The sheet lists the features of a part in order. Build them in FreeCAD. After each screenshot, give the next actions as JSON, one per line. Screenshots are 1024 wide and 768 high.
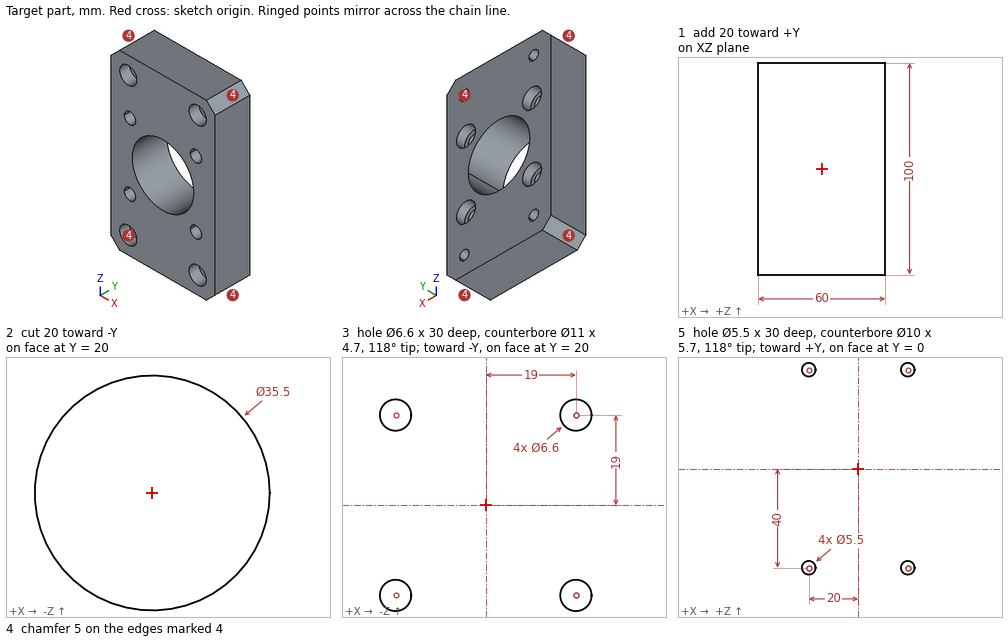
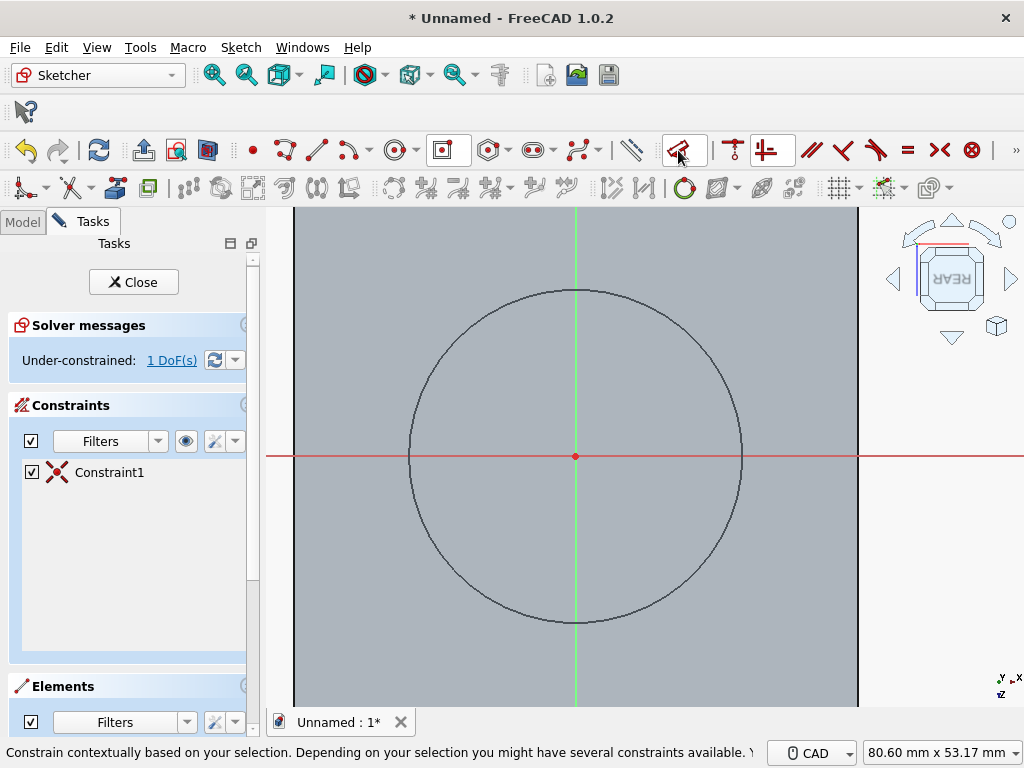
{"action": "left_click", "coordinate": [693, 338]}
{"action": "left_click", "coordinate": [716, 315]}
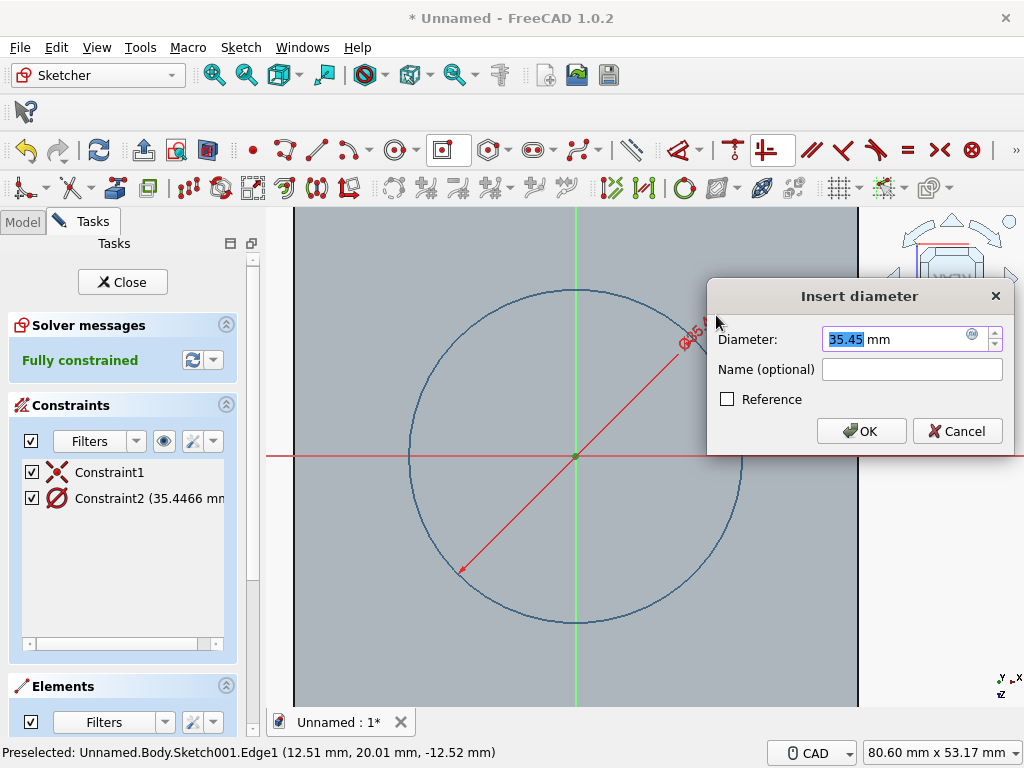
{"action": "type", "text": "35.5"}
{"action": "key", "text": "Return"}
{"action": "key", "text": "Escape"}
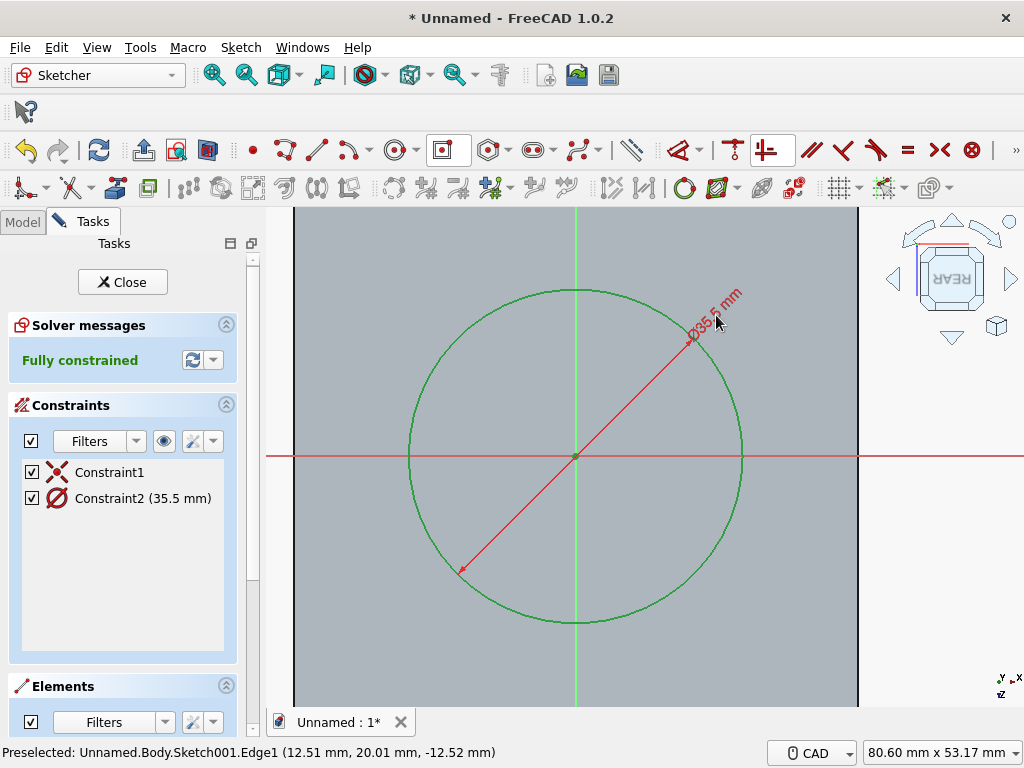
{"action": "left_click", "coordinate": [123, 282]}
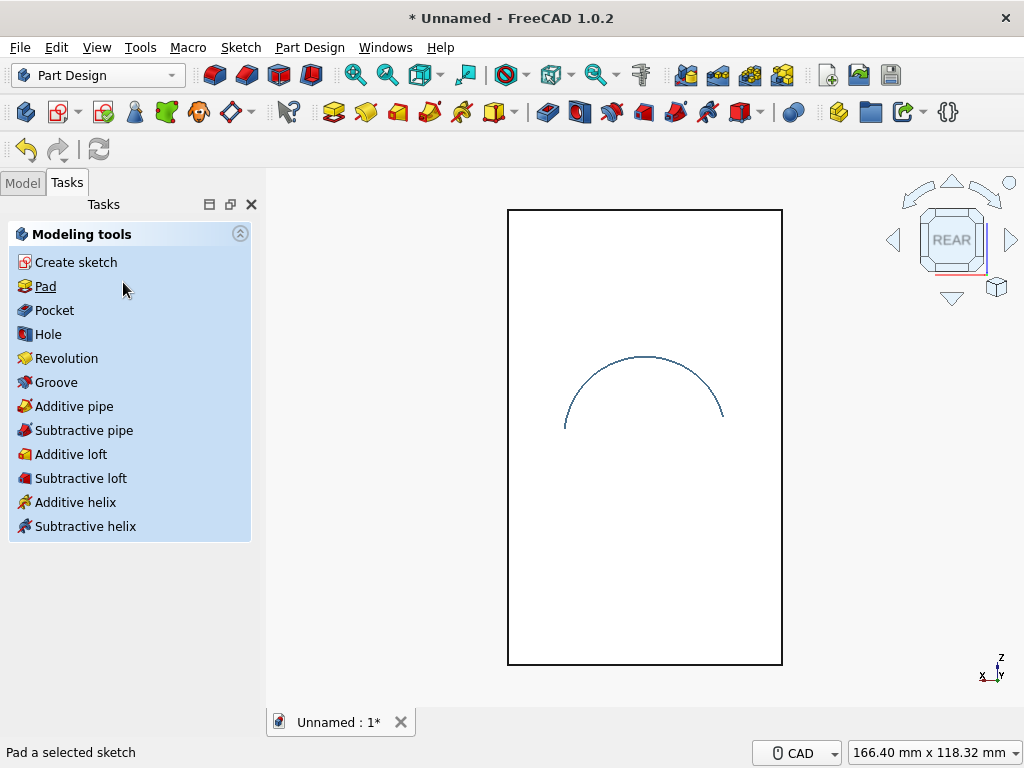
{"action": "left_click", "coordinate": [548, 112]}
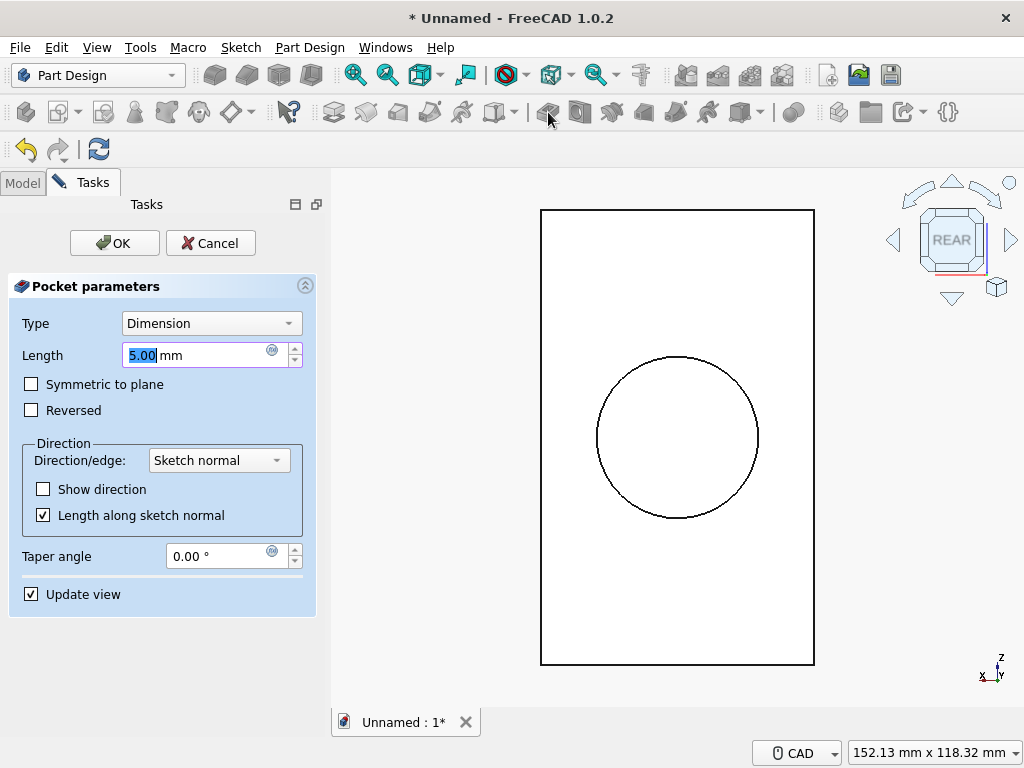
{"action": "type", "text": "20"}
{"action": "key", "text": "Tab"}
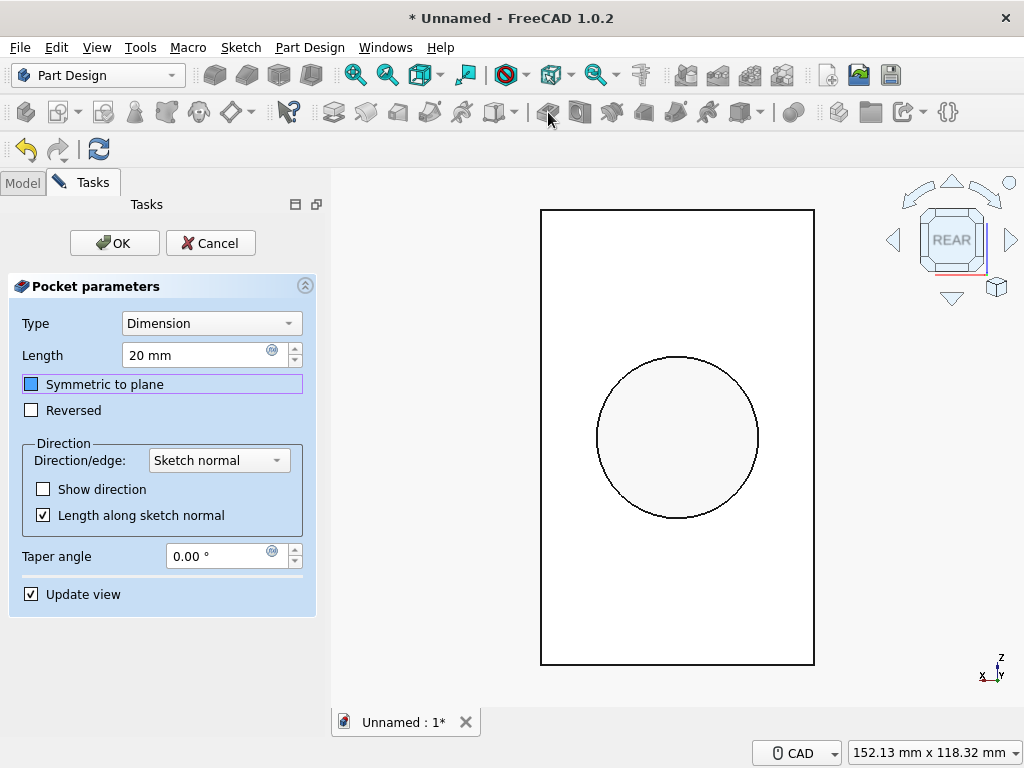
{"action": "left_click", "coordinate": [115, 243]}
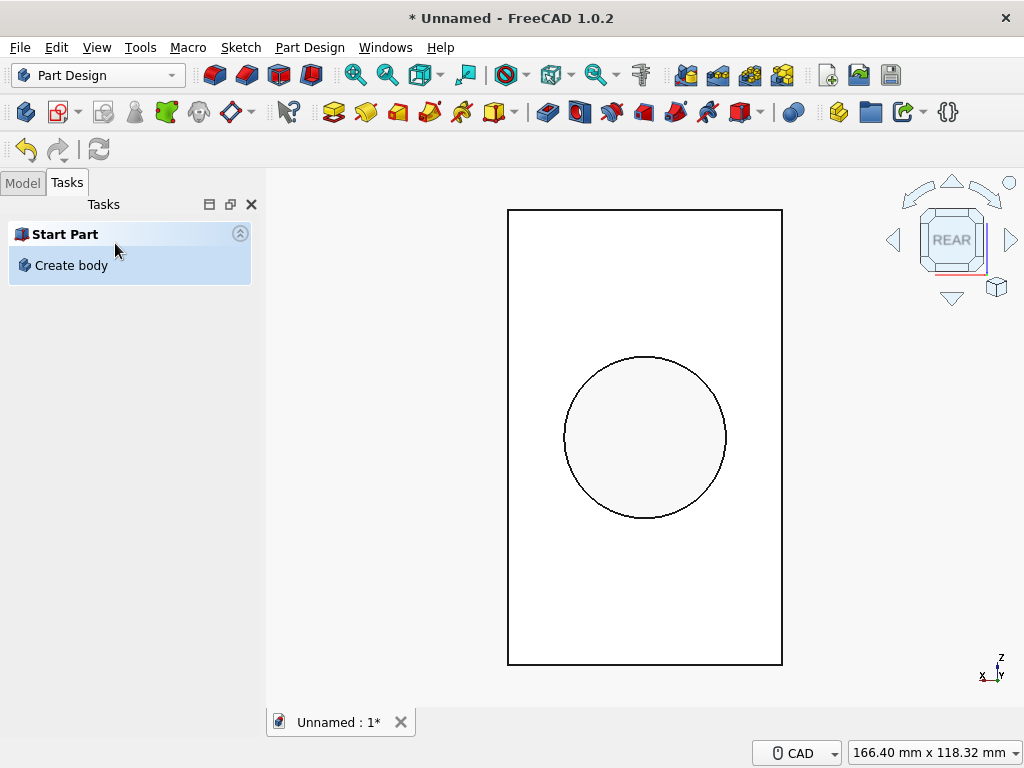
{"action": "left_click", "coordinate": [723, 306]}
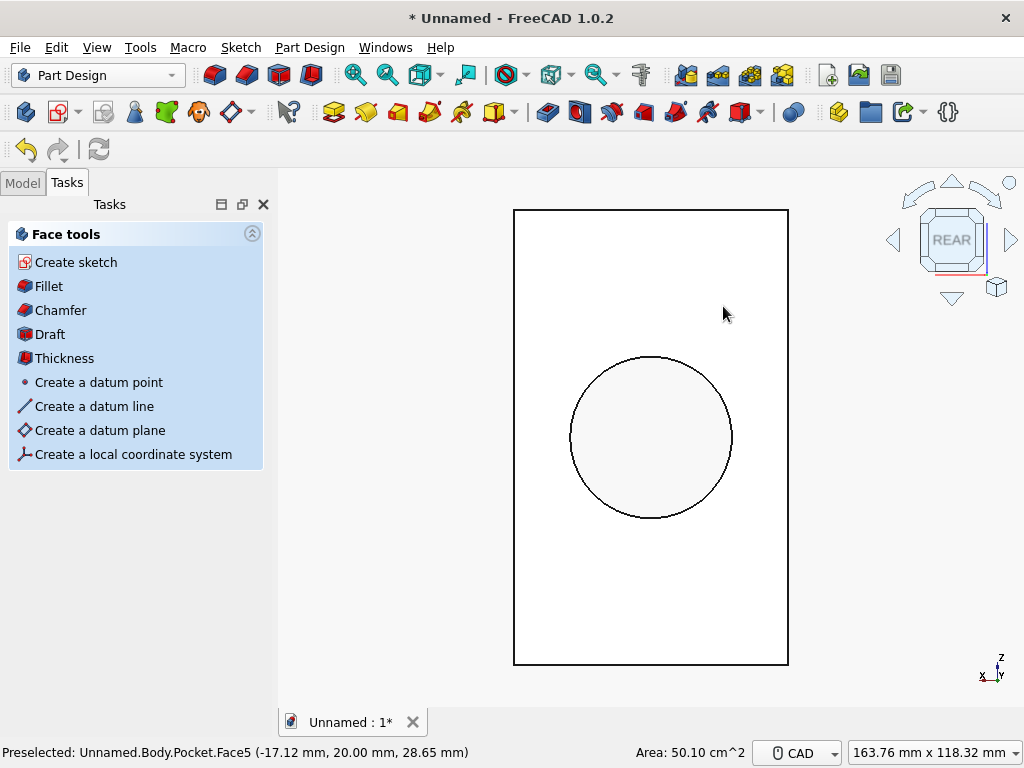
{"action": "left_click", "coordinate": [58, 112]}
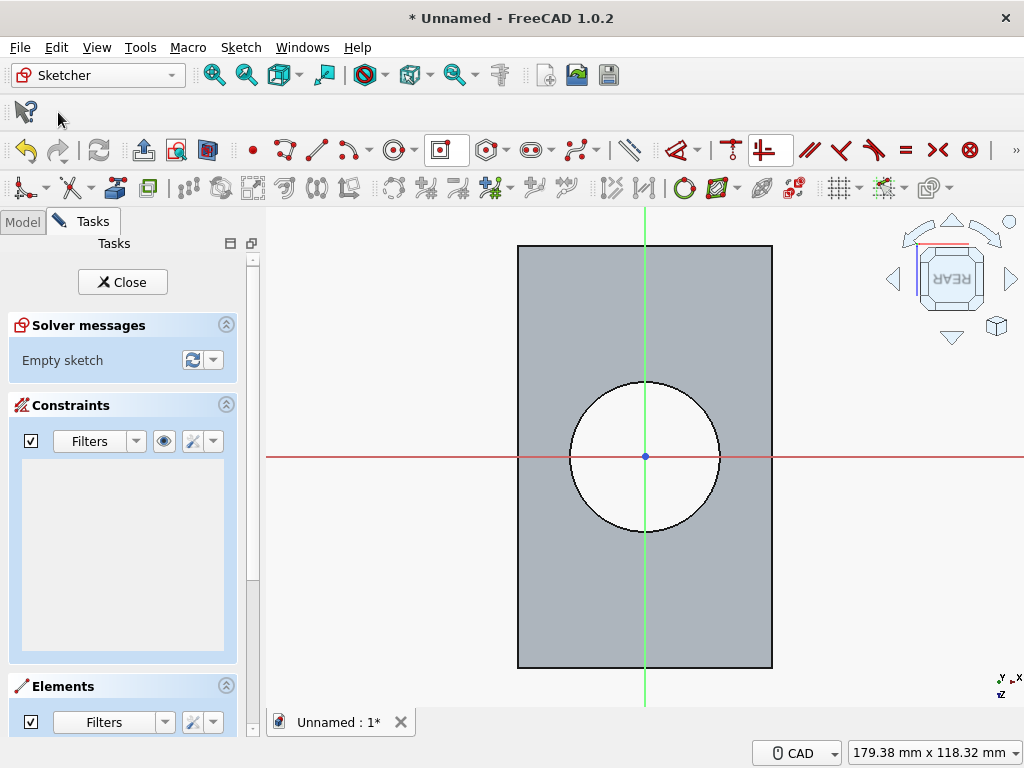
{"action": "scroll", "coordinate": [728, 457], "scroll_direction": "up", "scroll_amount": 3}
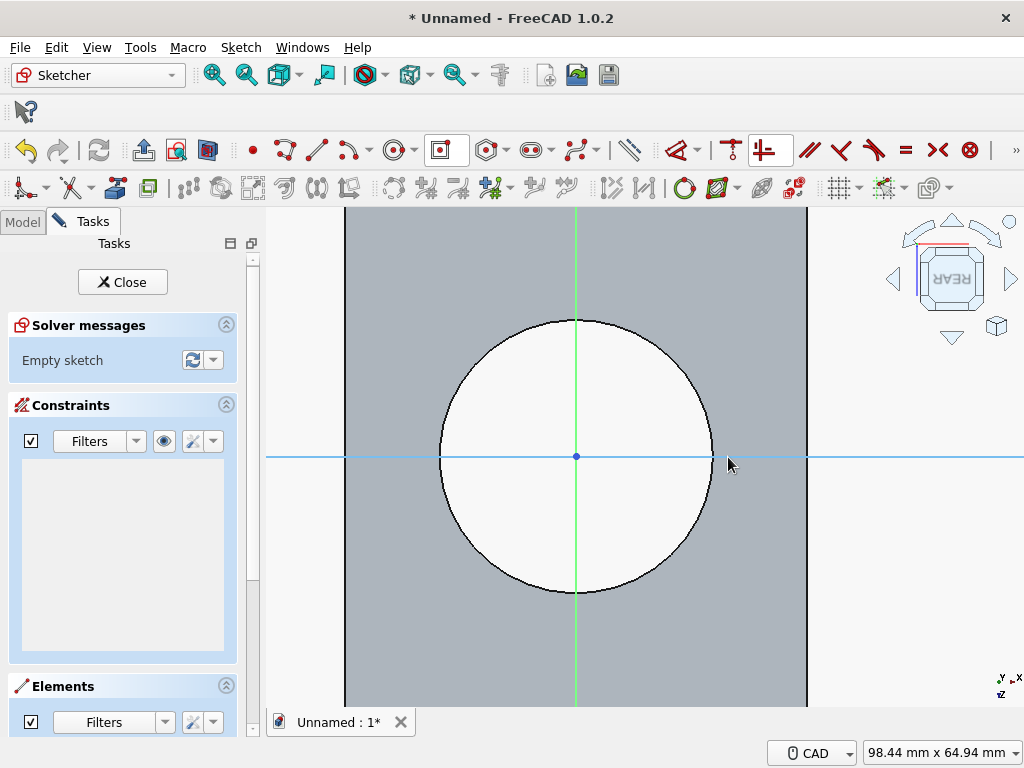
{"action": "left_click", "coordinate": [394, 150]}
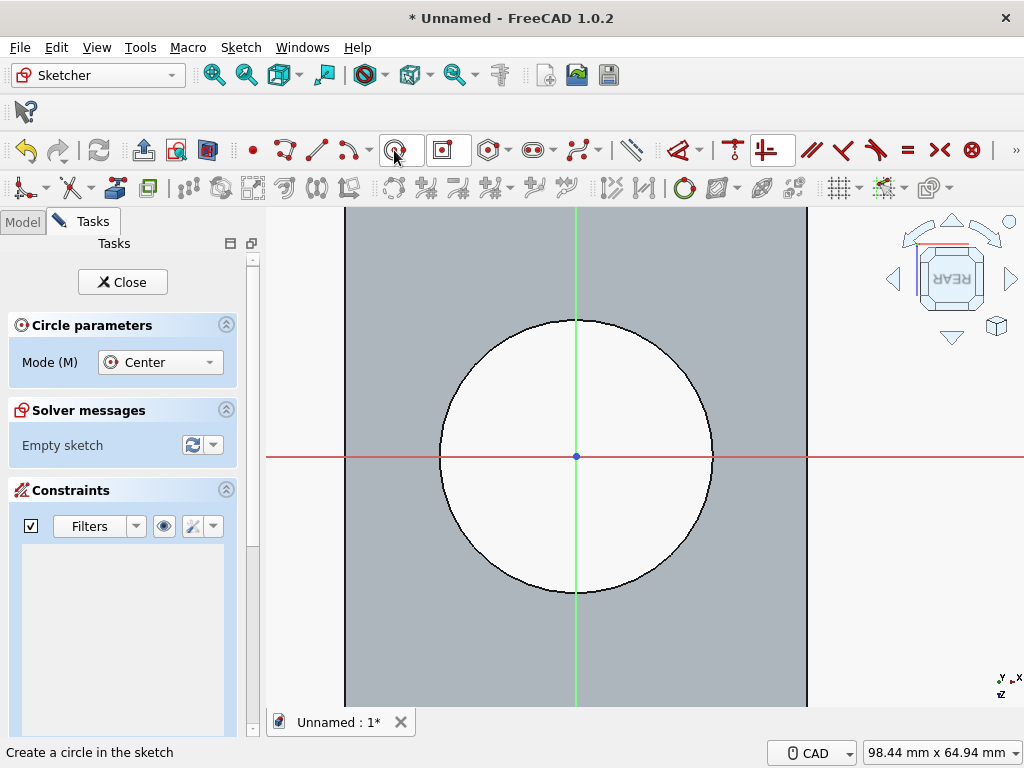
{"action": "left_click", "coordinate": [723, 310]}
{"action": "left_click", "coordinate": [741, 292]}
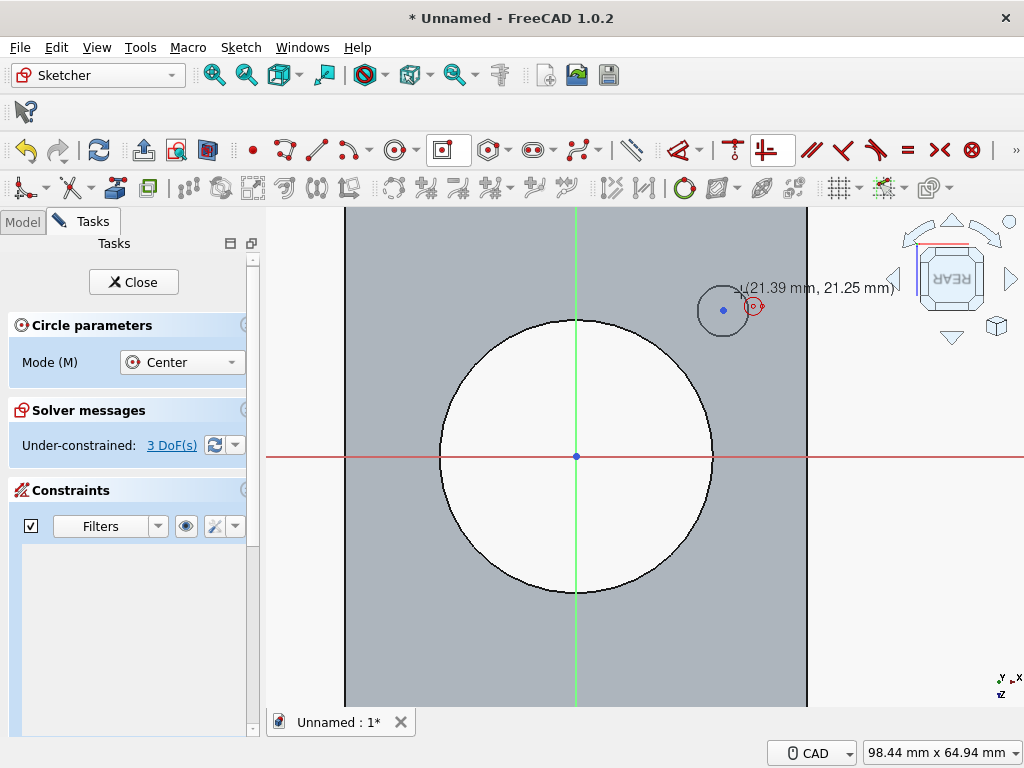
{"action": "left_click", "coordinate": [723, 603]}
{"action": "left_click", "coordinate": [741, 585]}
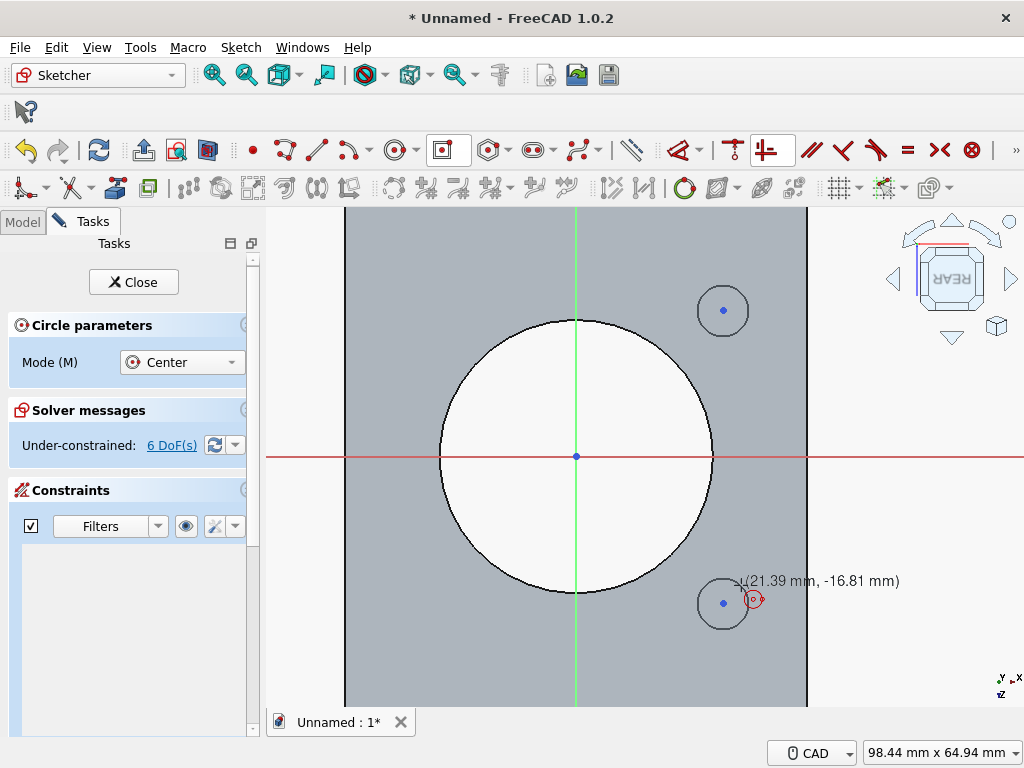
{"action": "left_click", "coordinate": [430, 310]}
{"action": "left_click", "coordinate": [448, 292]}